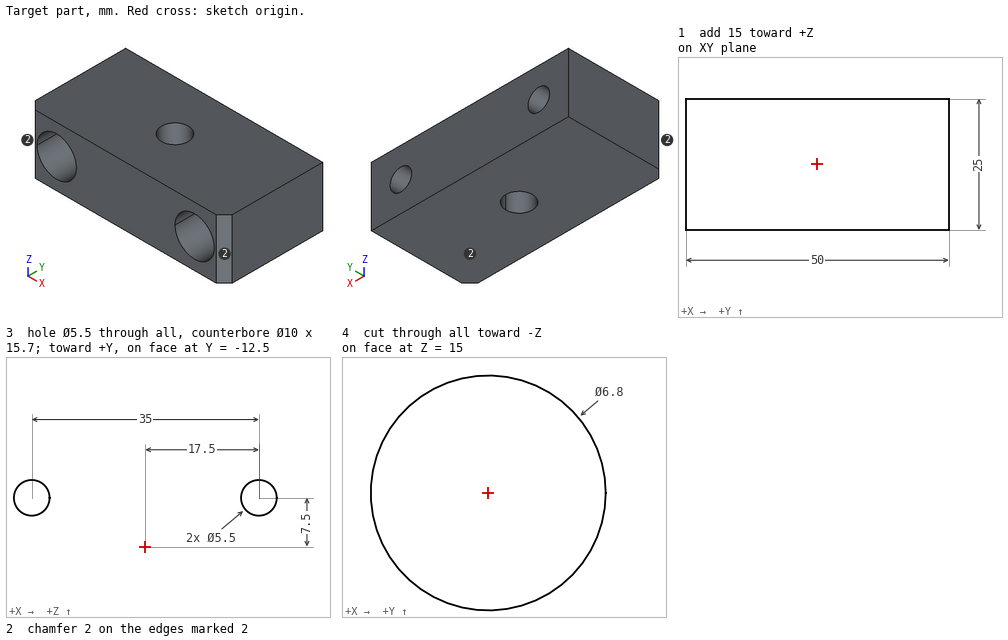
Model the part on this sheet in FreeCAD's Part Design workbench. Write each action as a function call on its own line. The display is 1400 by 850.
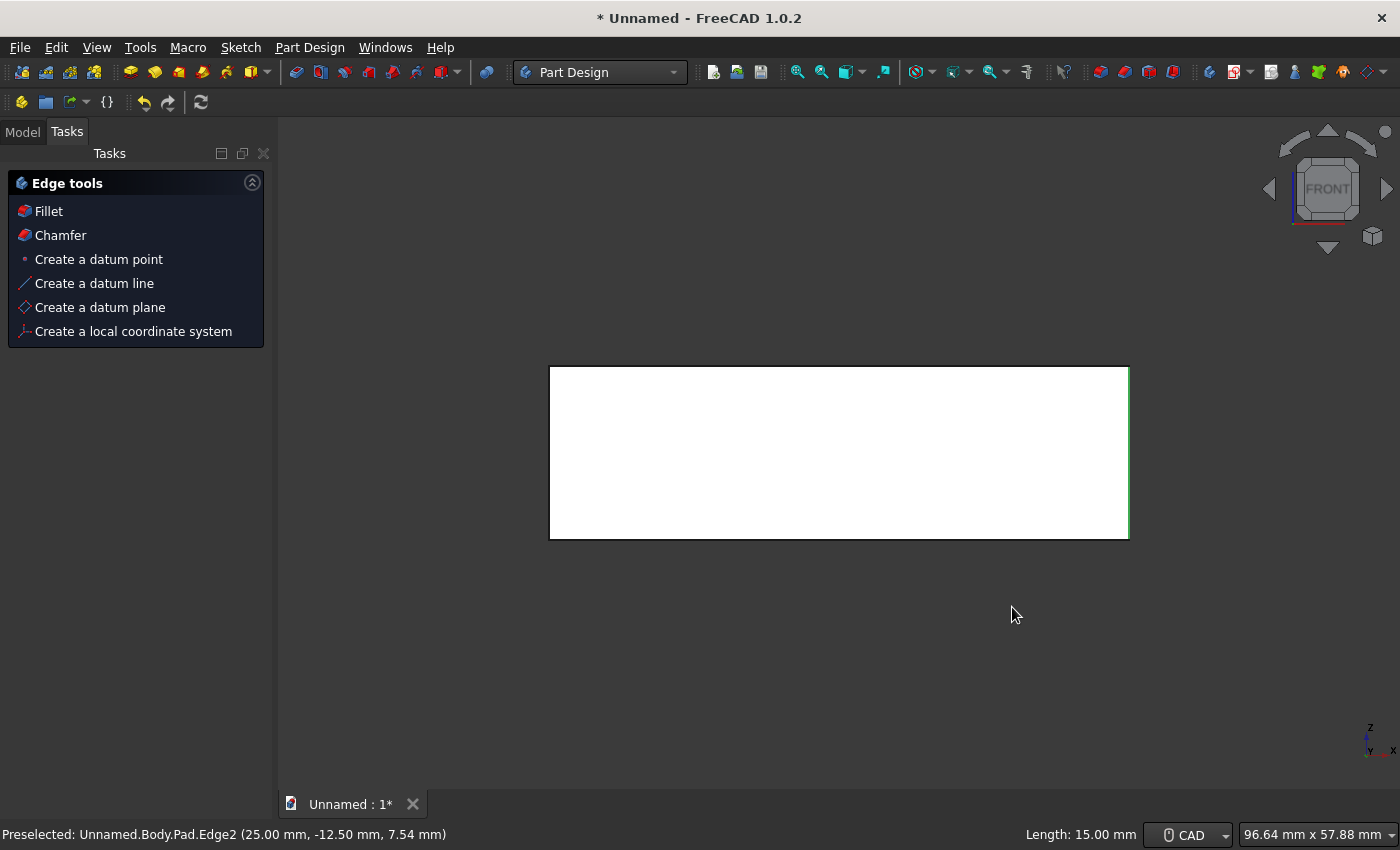
click(549, 452, ctrl)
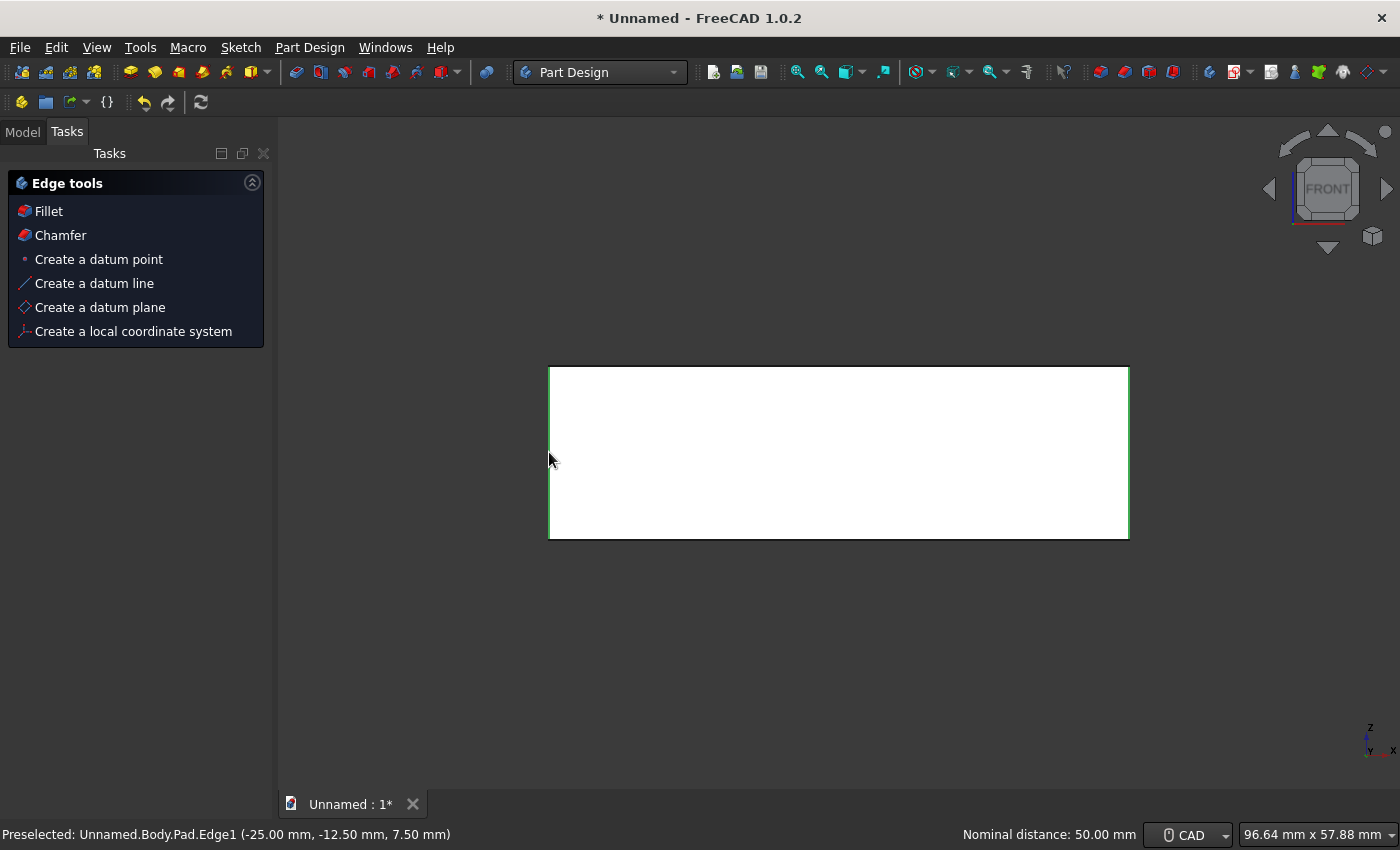
click(1126, 72)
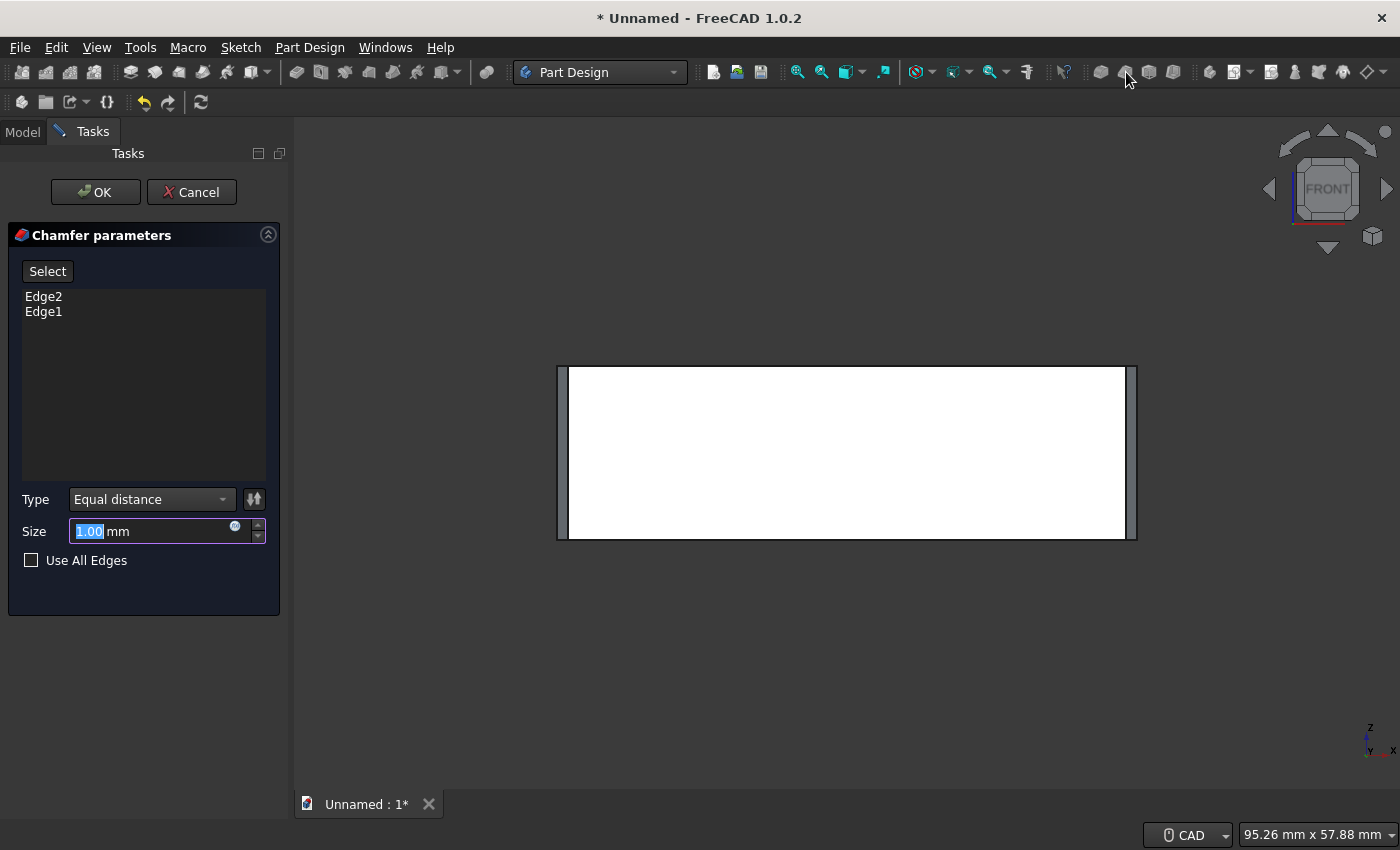
text(2)
key(Tab)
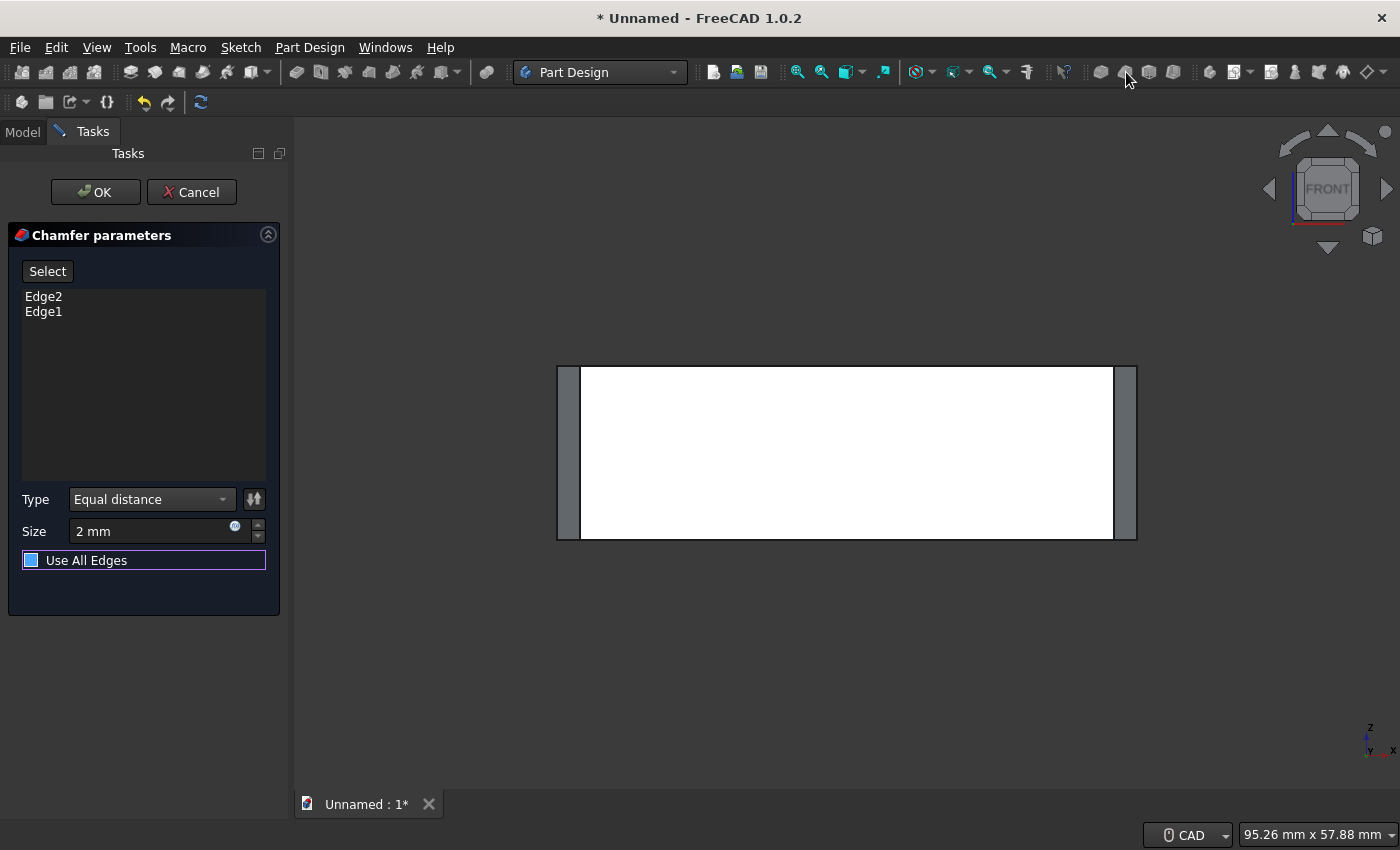
click(96, 192)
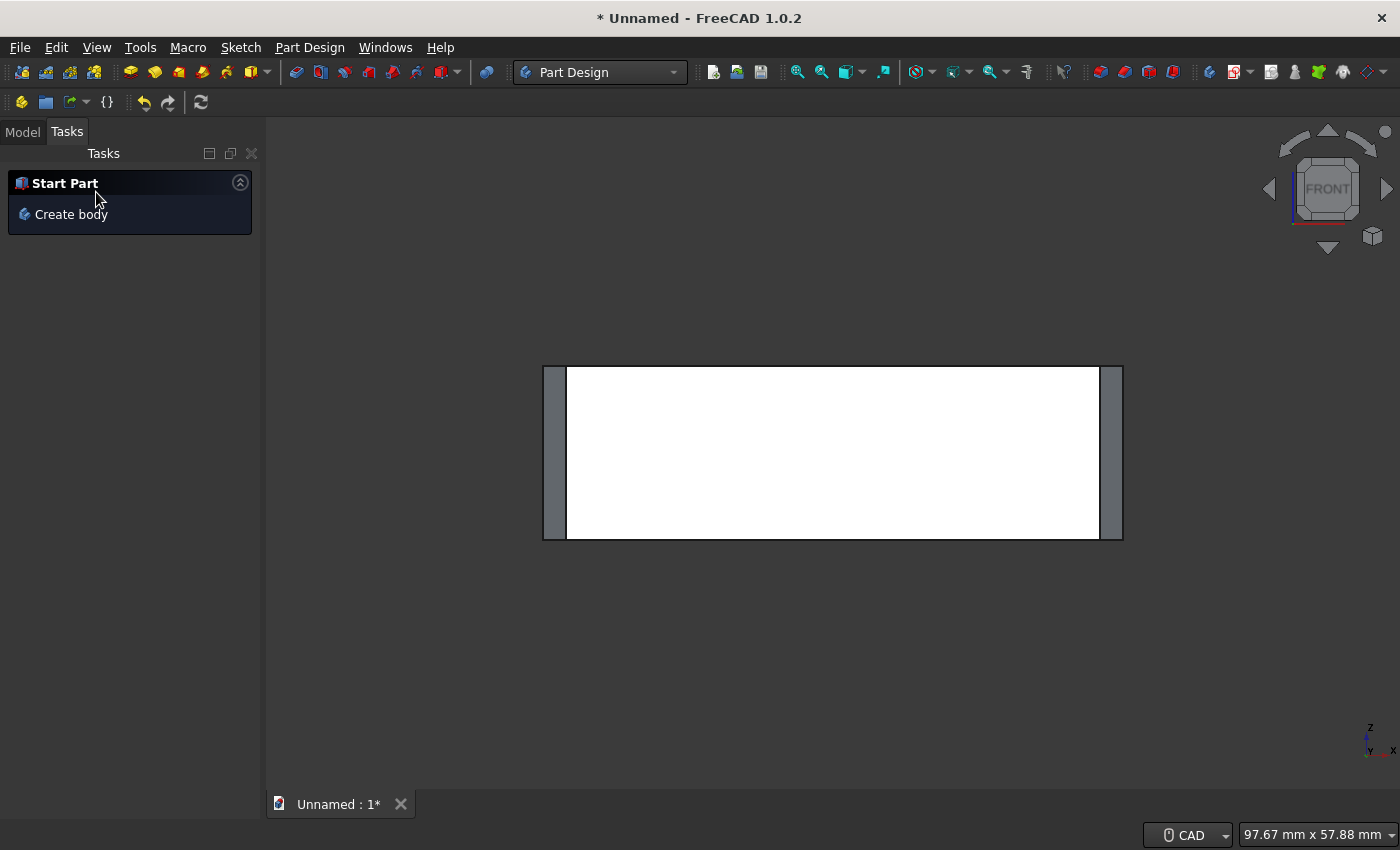
click(986, 452)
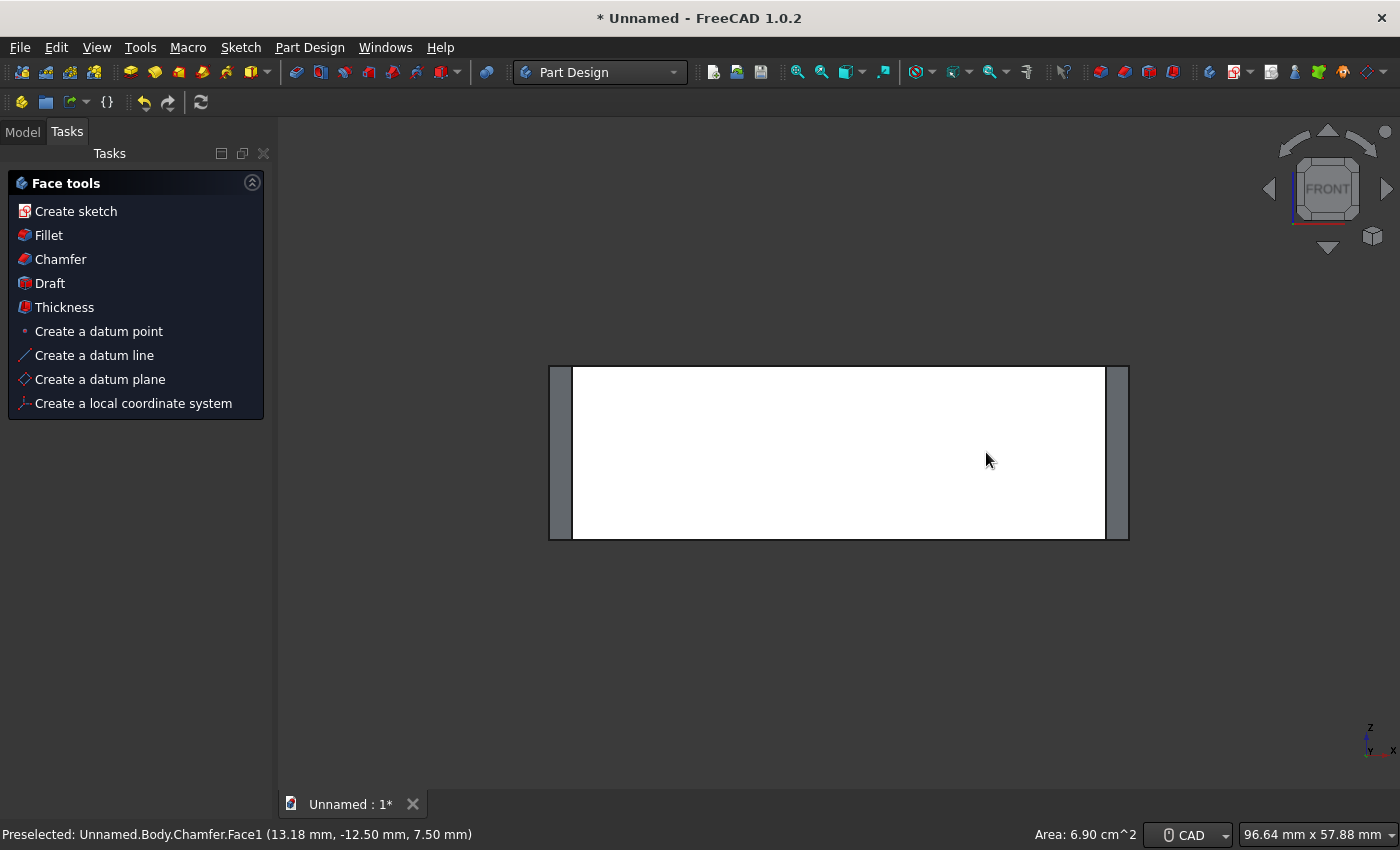
click(1234, 72)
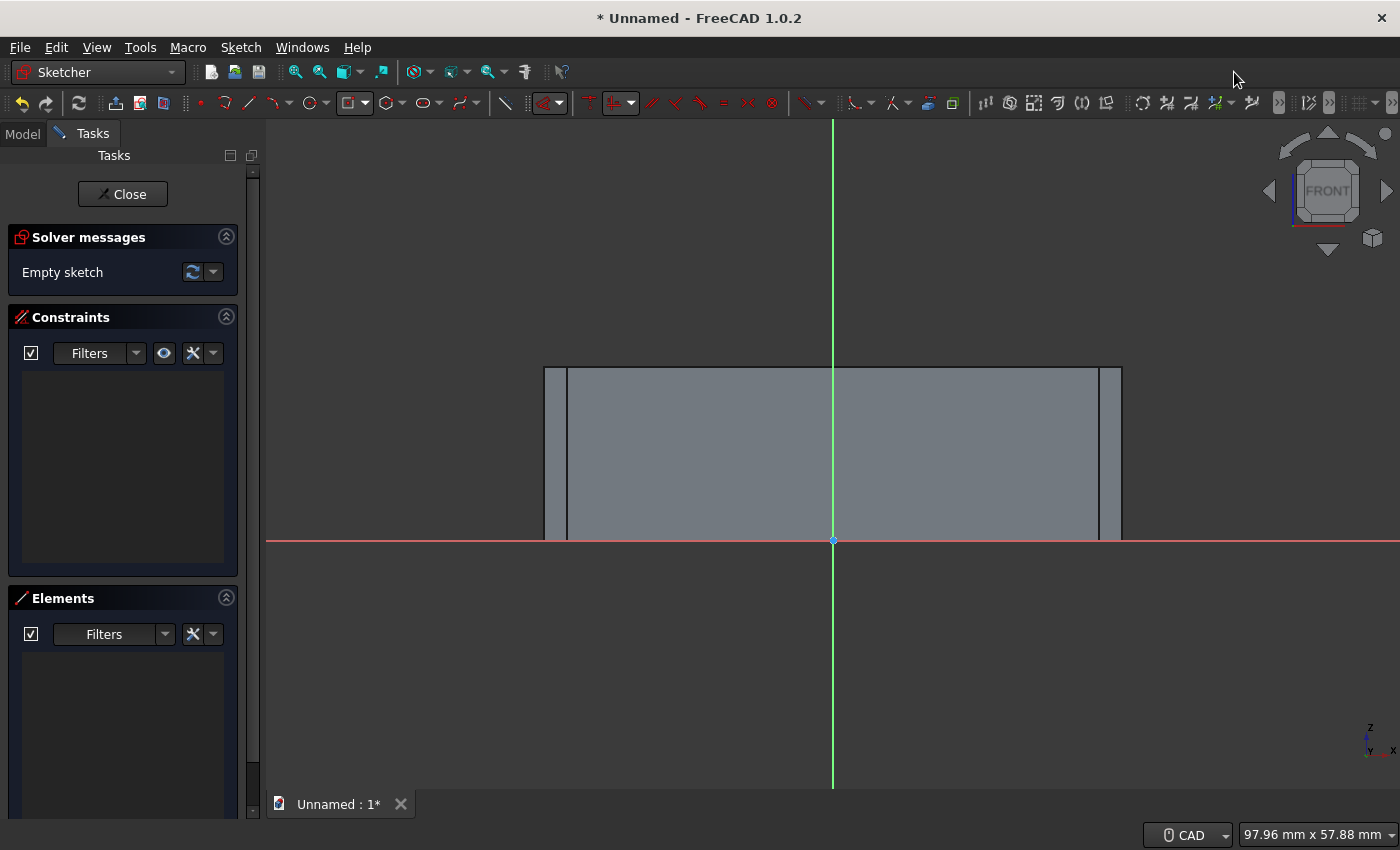
scroll(972, 537, up, 2)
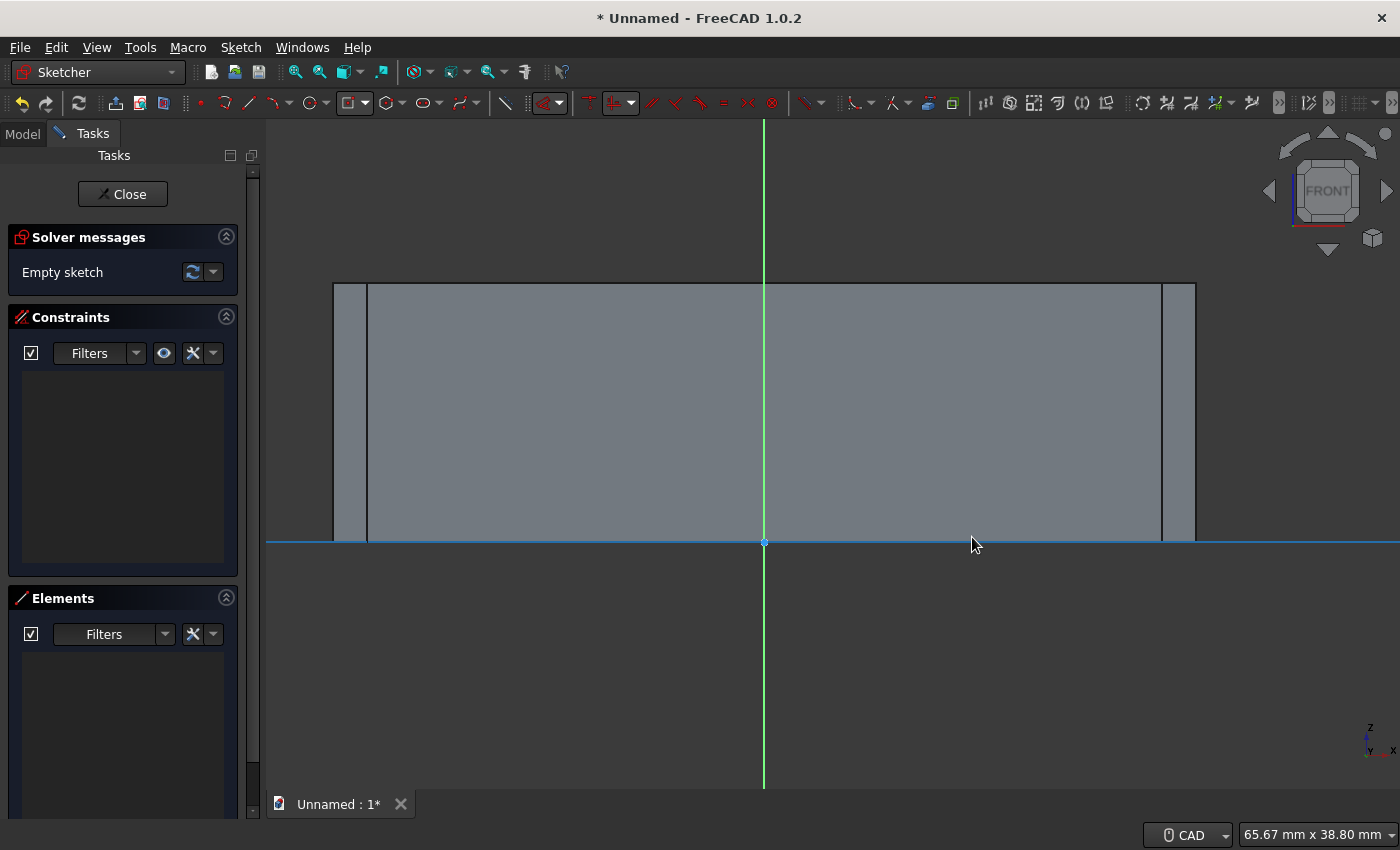
click(310, 104)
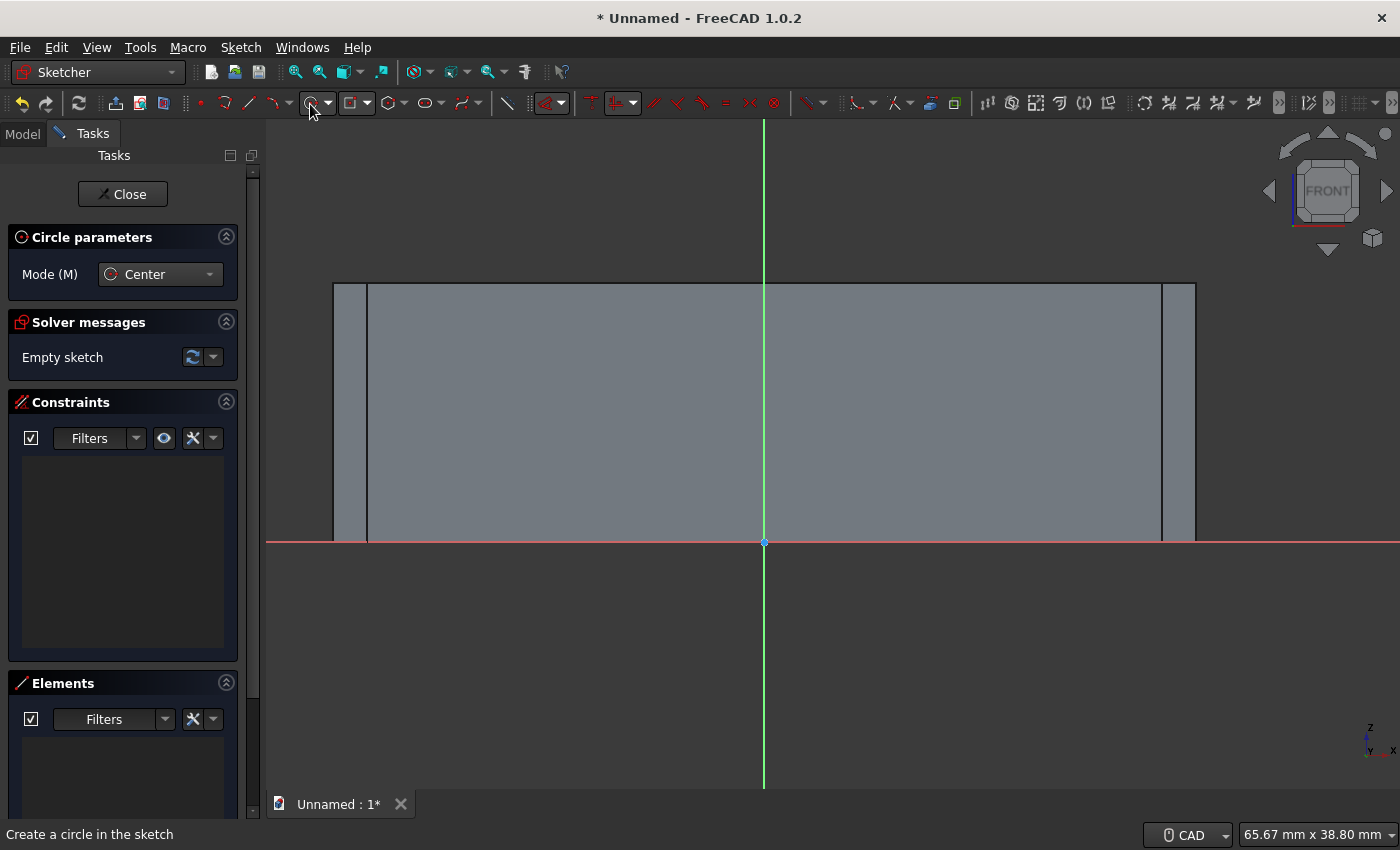
click(1067, 413)
move(1100, 379)